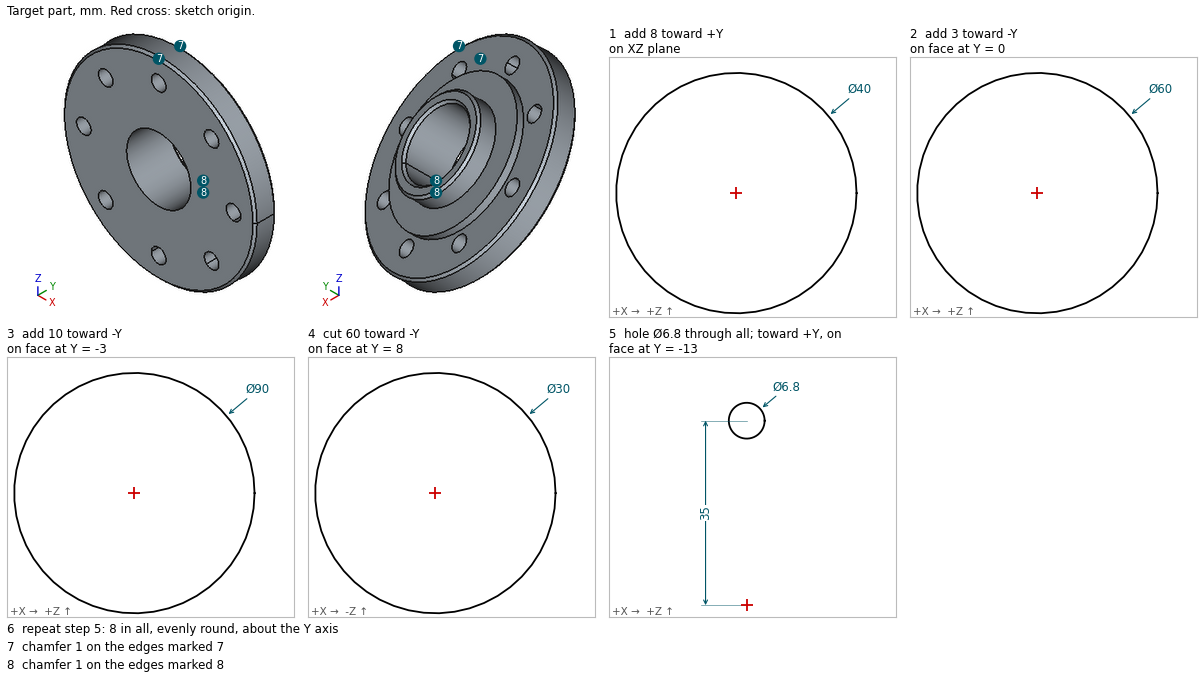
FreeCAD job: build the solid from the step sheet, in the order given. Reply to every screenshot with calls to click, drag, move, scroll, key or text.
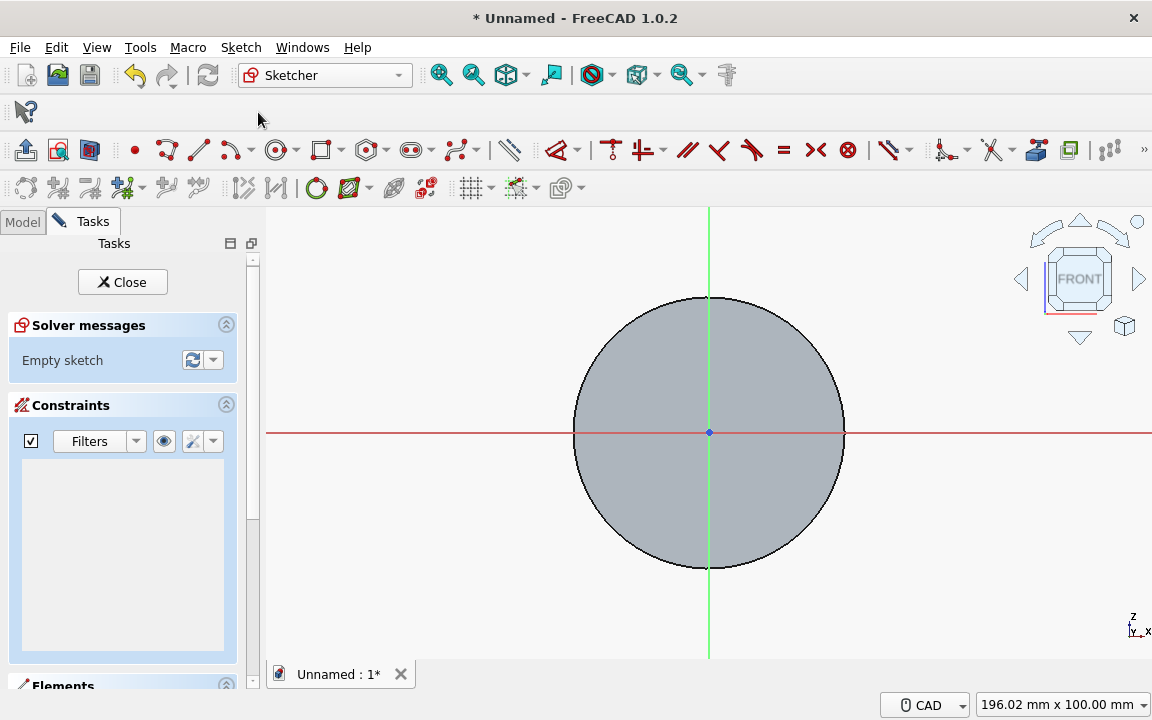
scroll(501, 433, down, 2)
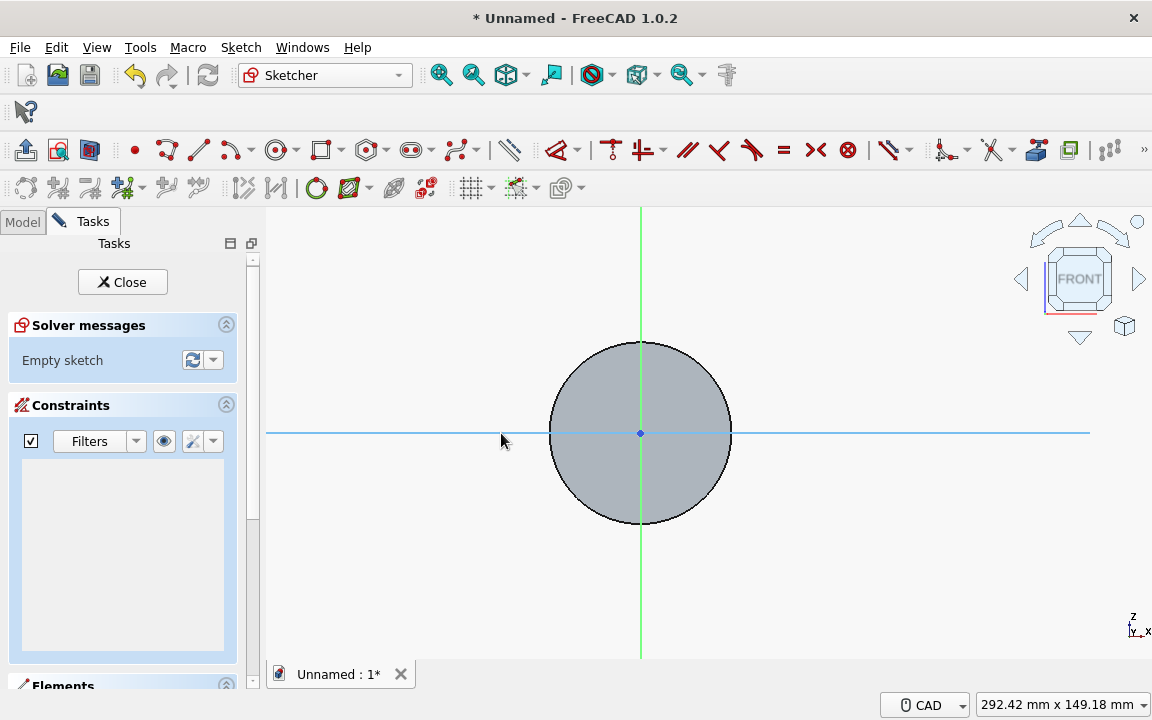
click(276, 150)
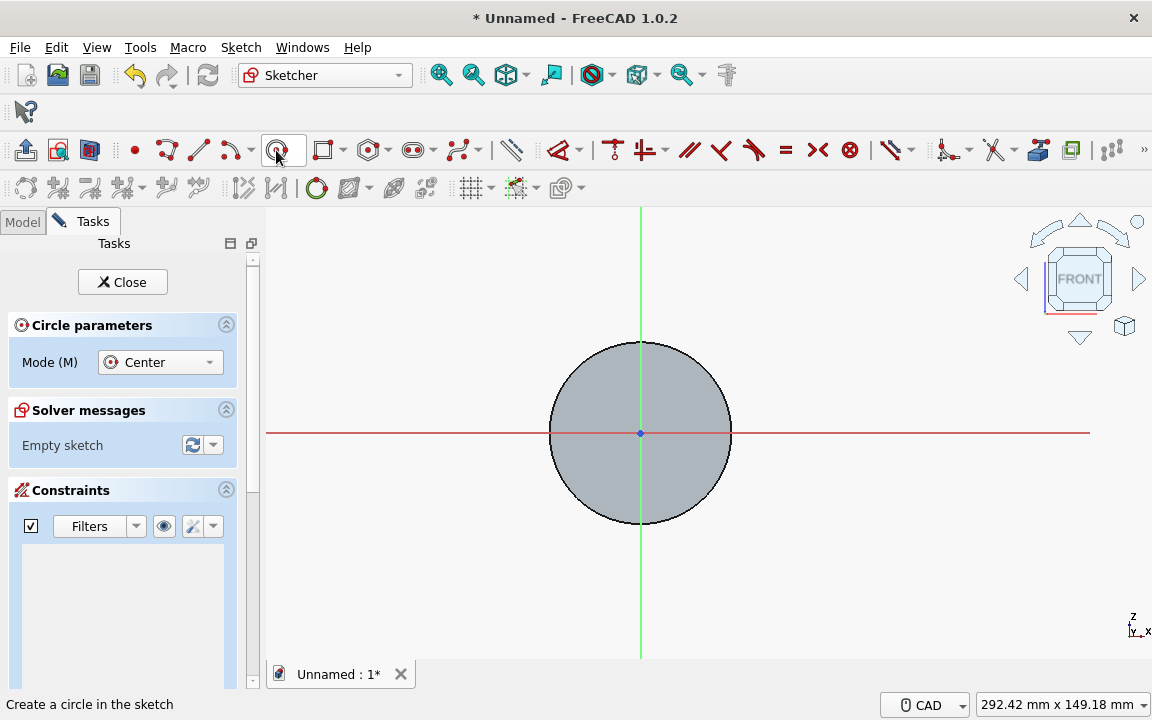
click(641, 433)
move(737, 337)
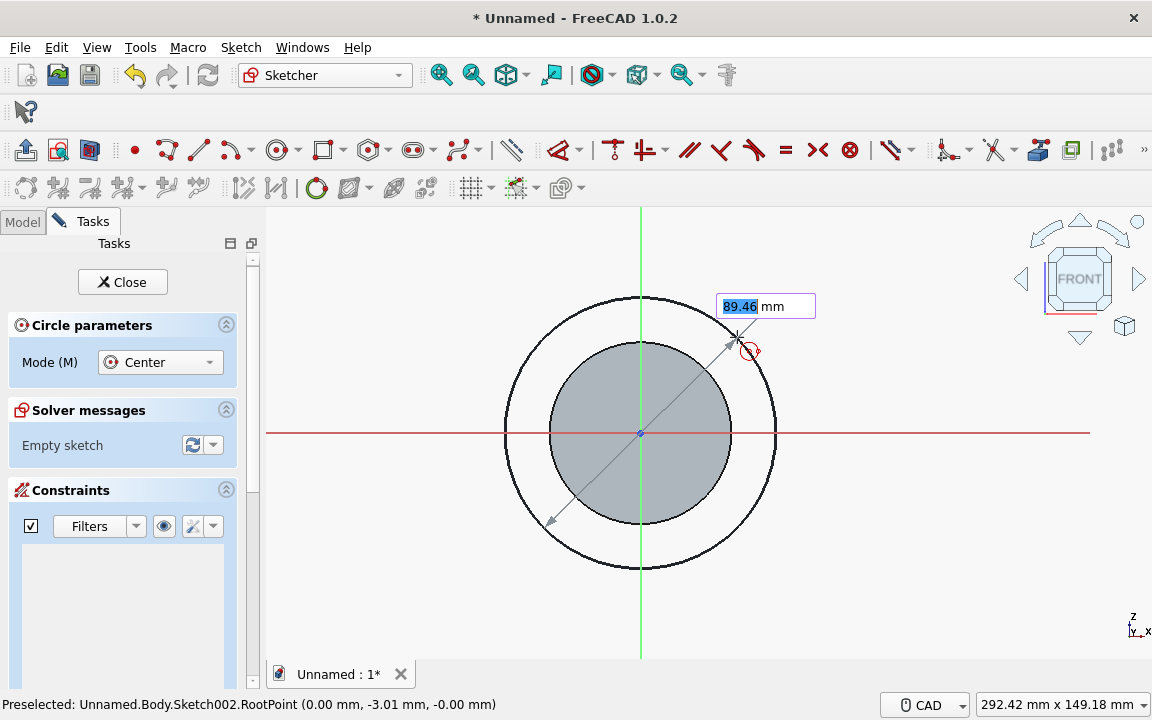
text(90)
key(Return)
key(Escape)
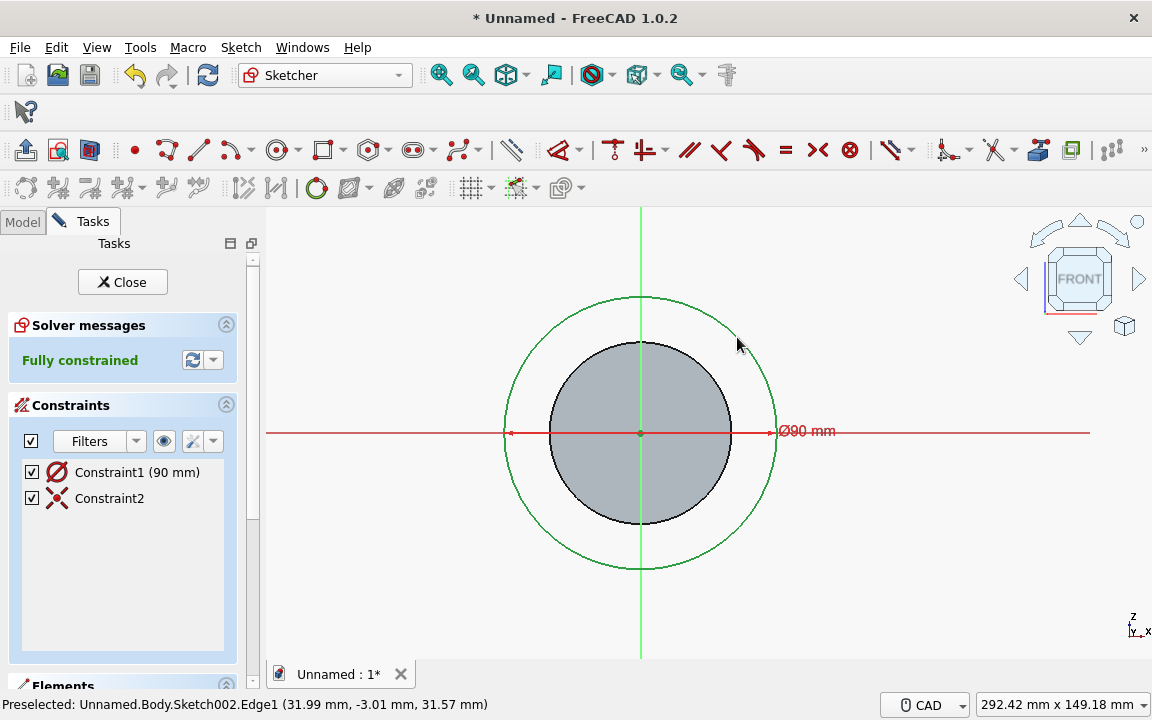
click(123, 282)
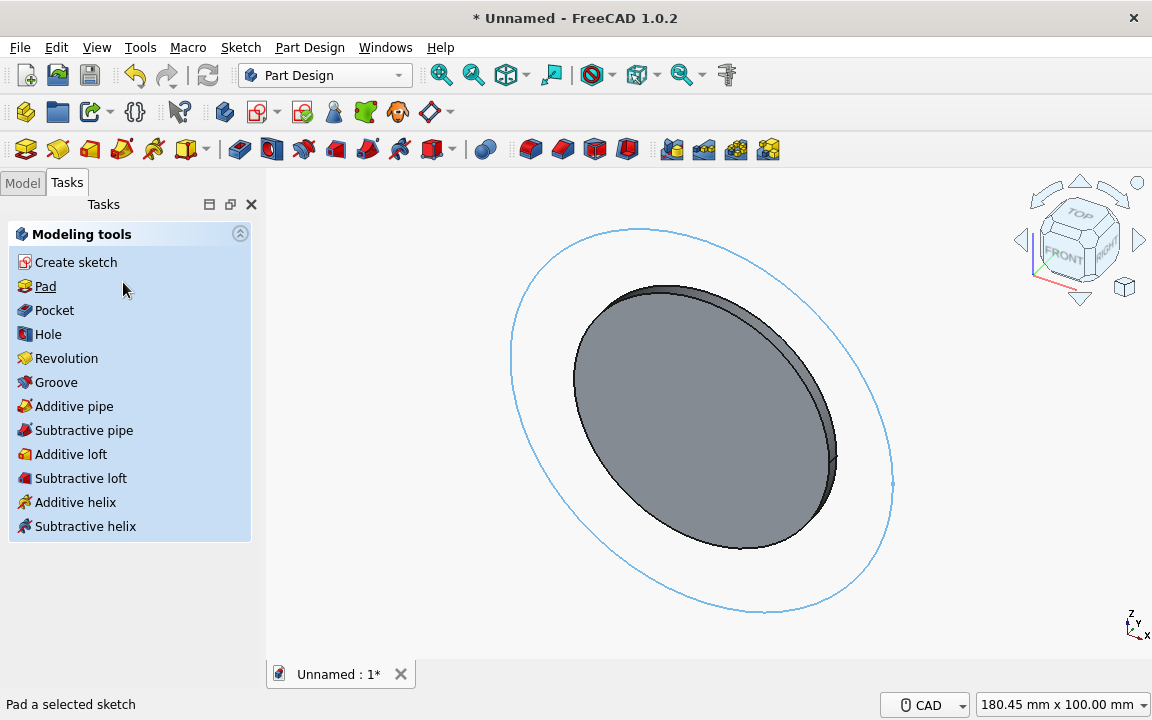
click(26, 150)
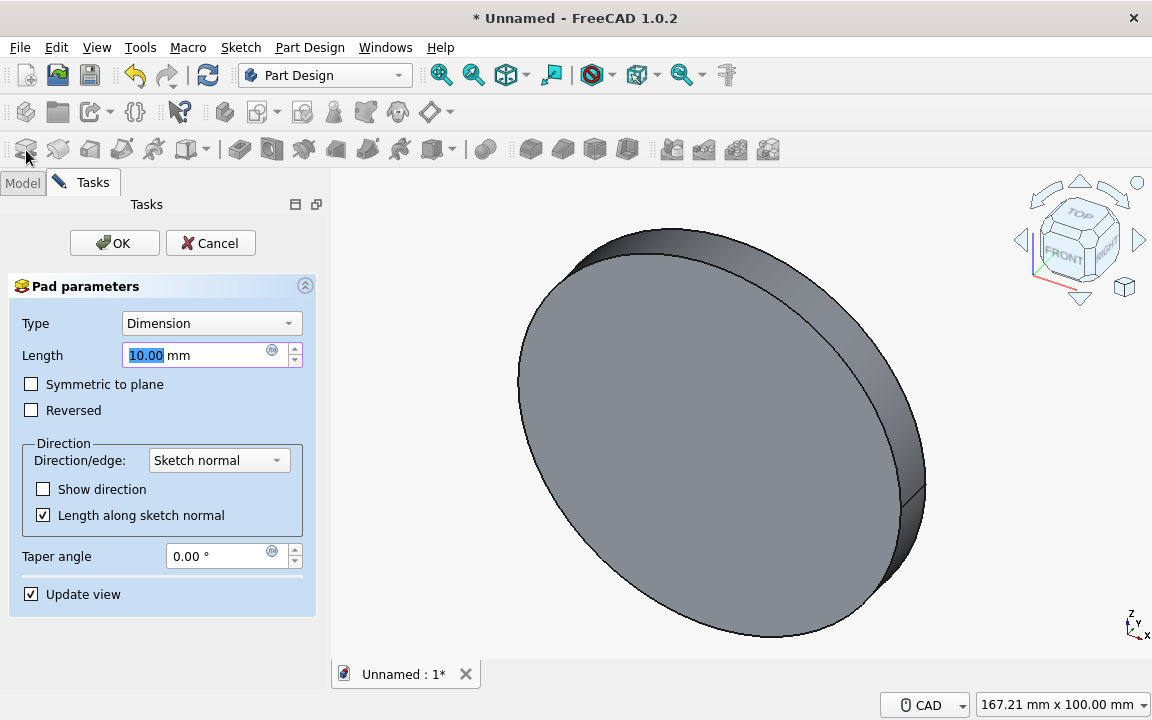
text(10)
key(Tab)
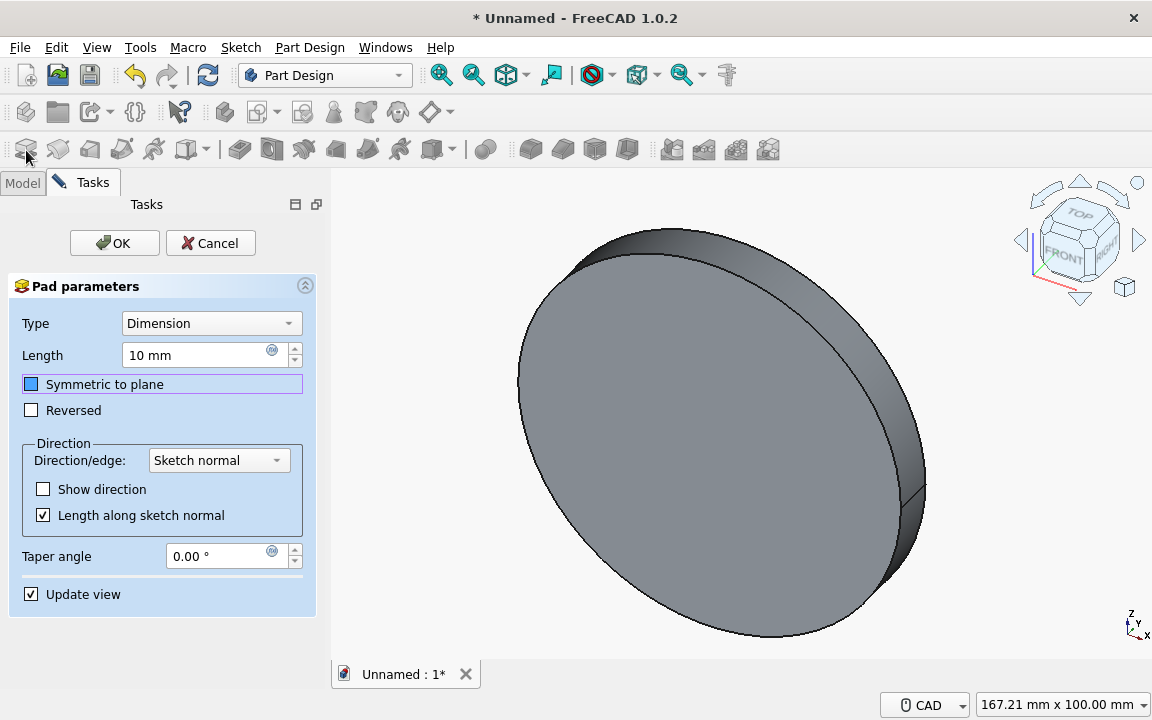
click(115, 243)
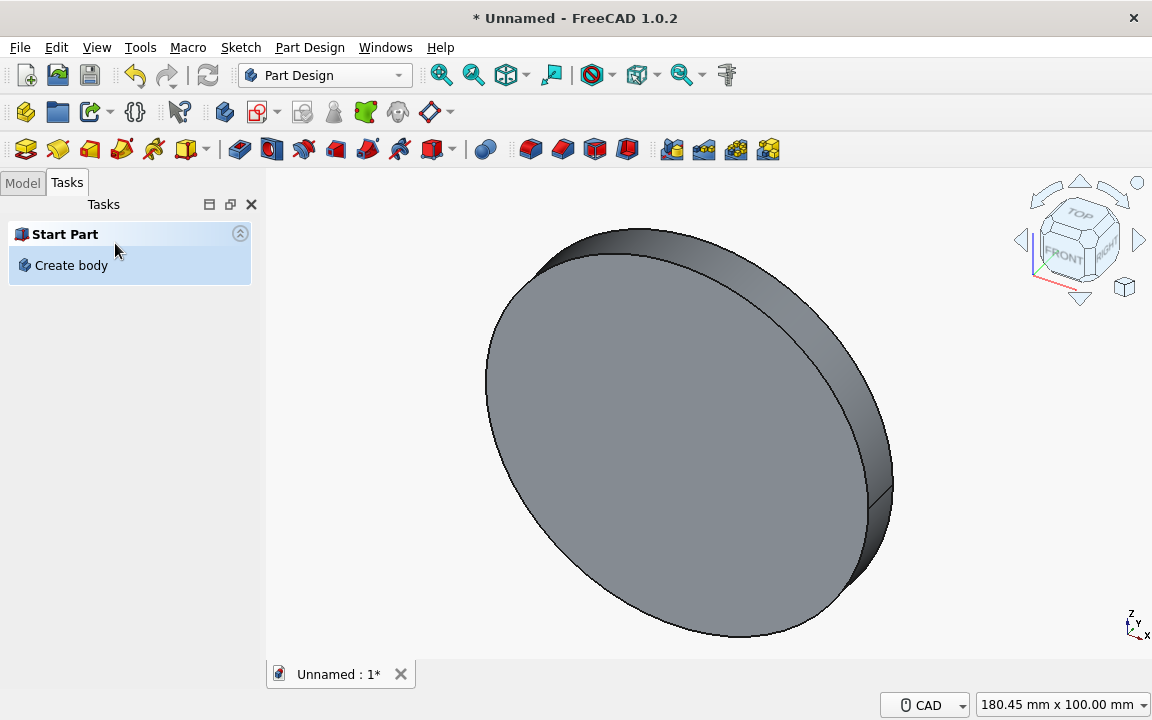
click(442, 76)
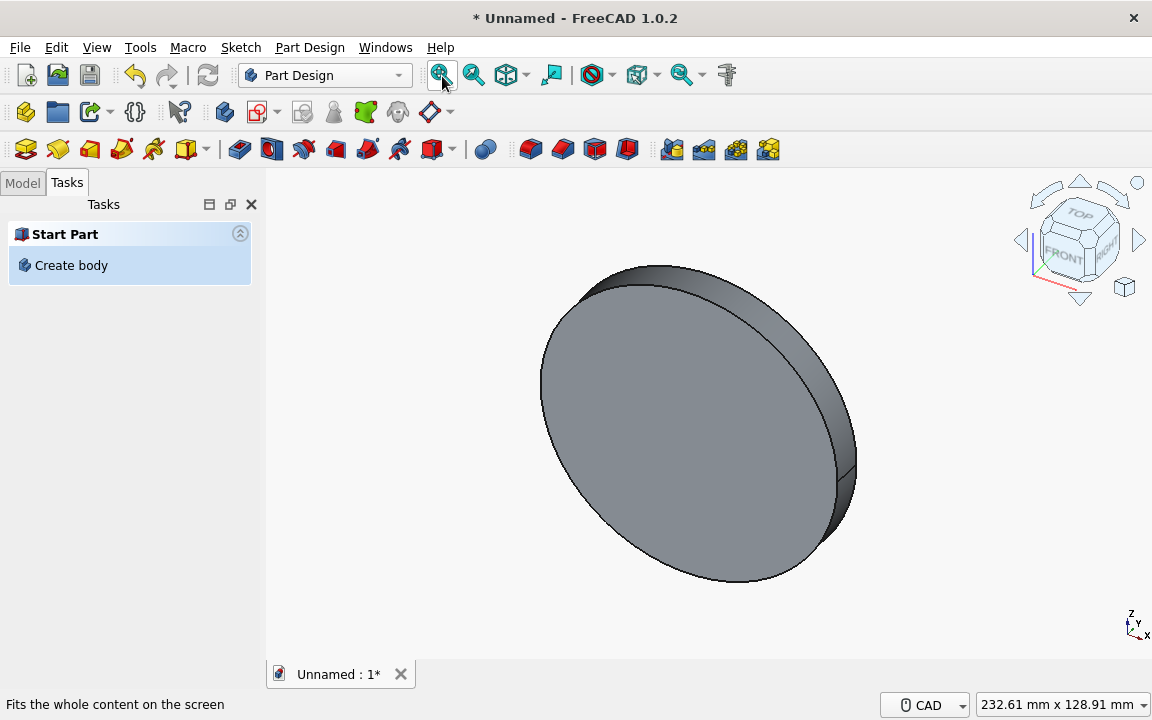
key(4)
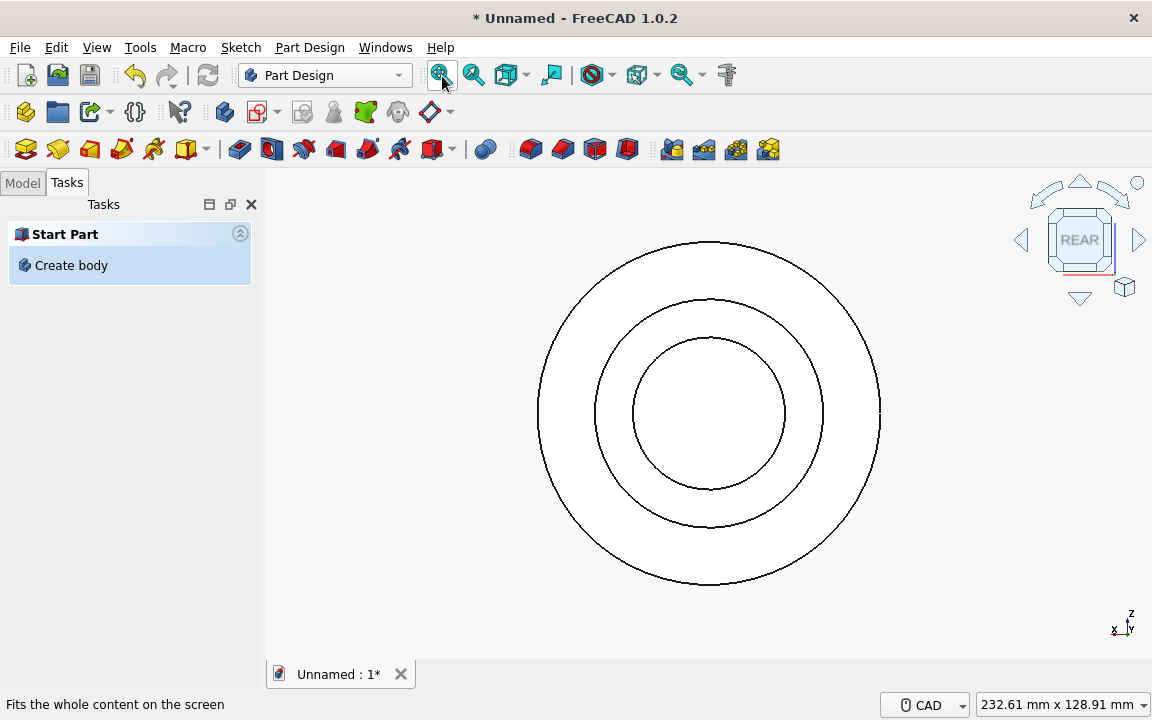
click(709, 412)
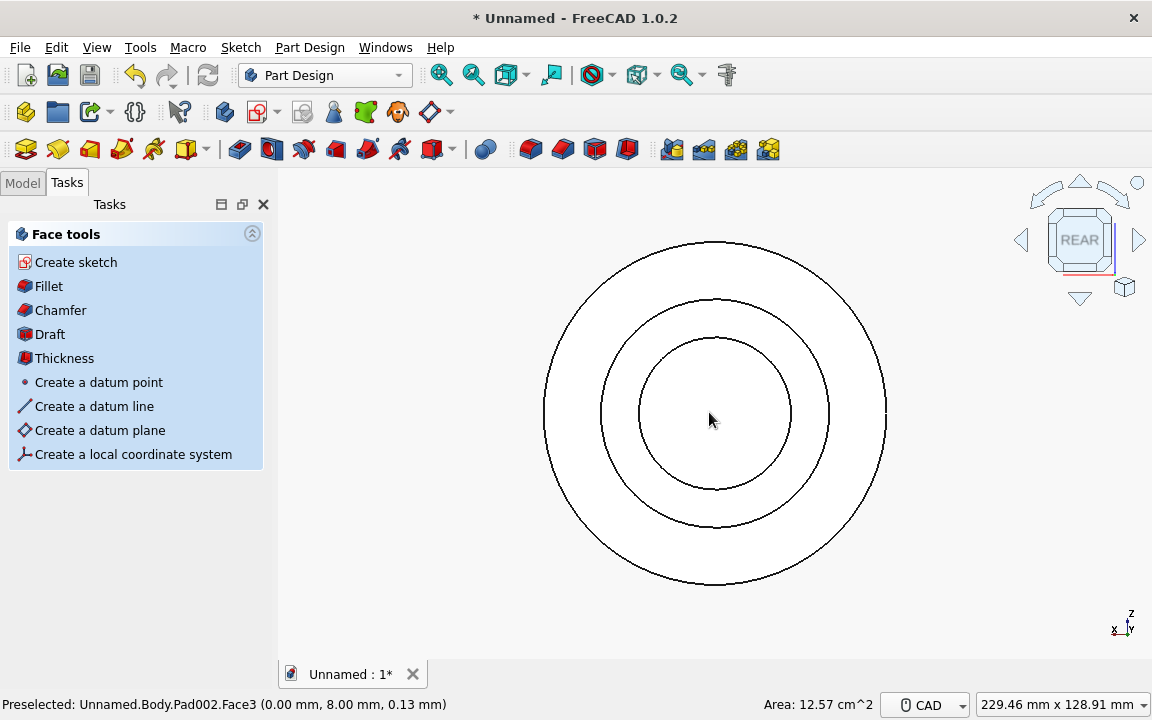
click(258, 112)